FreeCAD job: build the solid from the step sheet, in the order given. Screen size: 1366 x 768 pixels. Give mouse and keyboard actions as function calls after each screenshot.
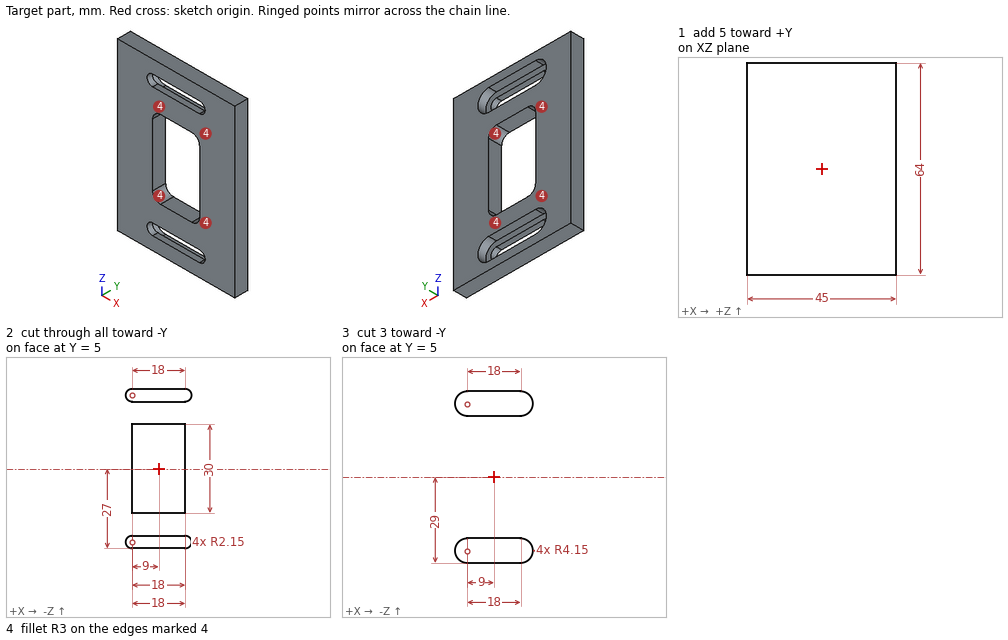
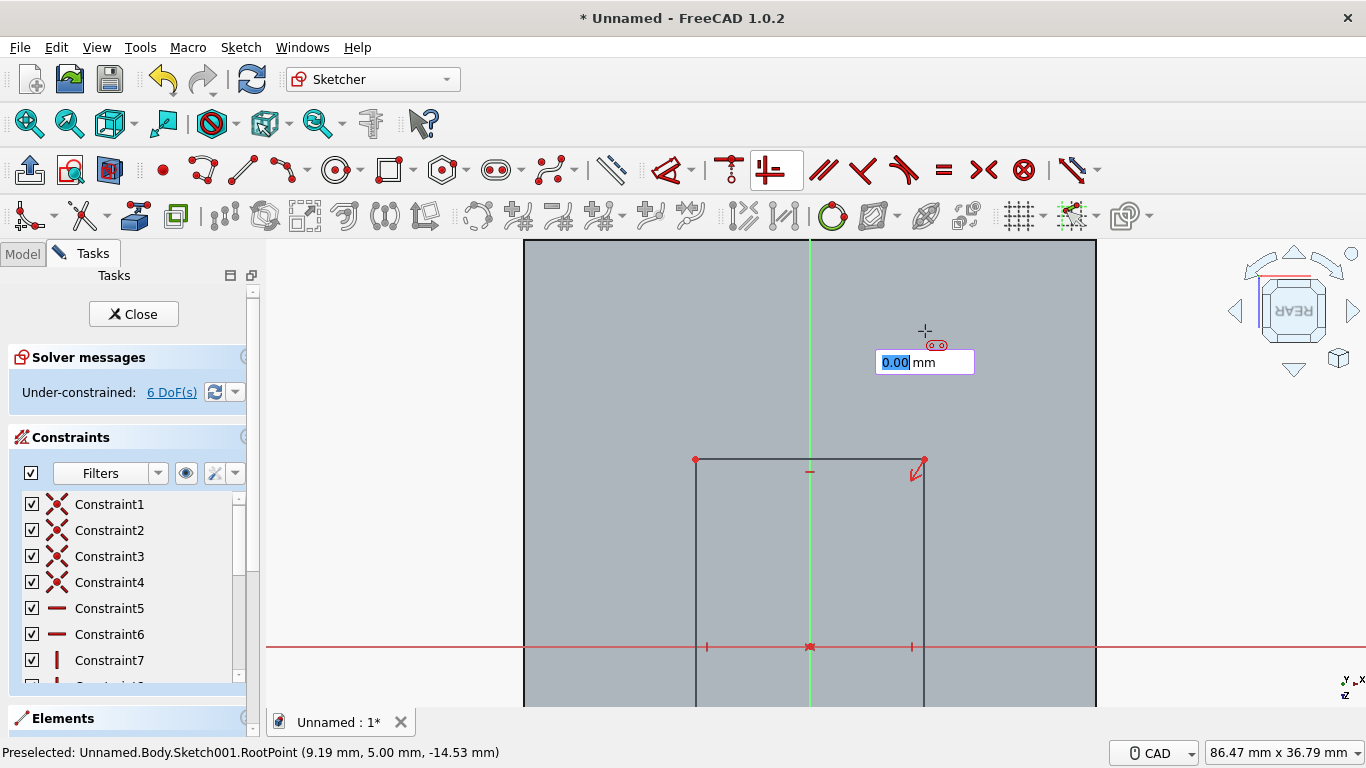
click(776, 358)
key(Escape)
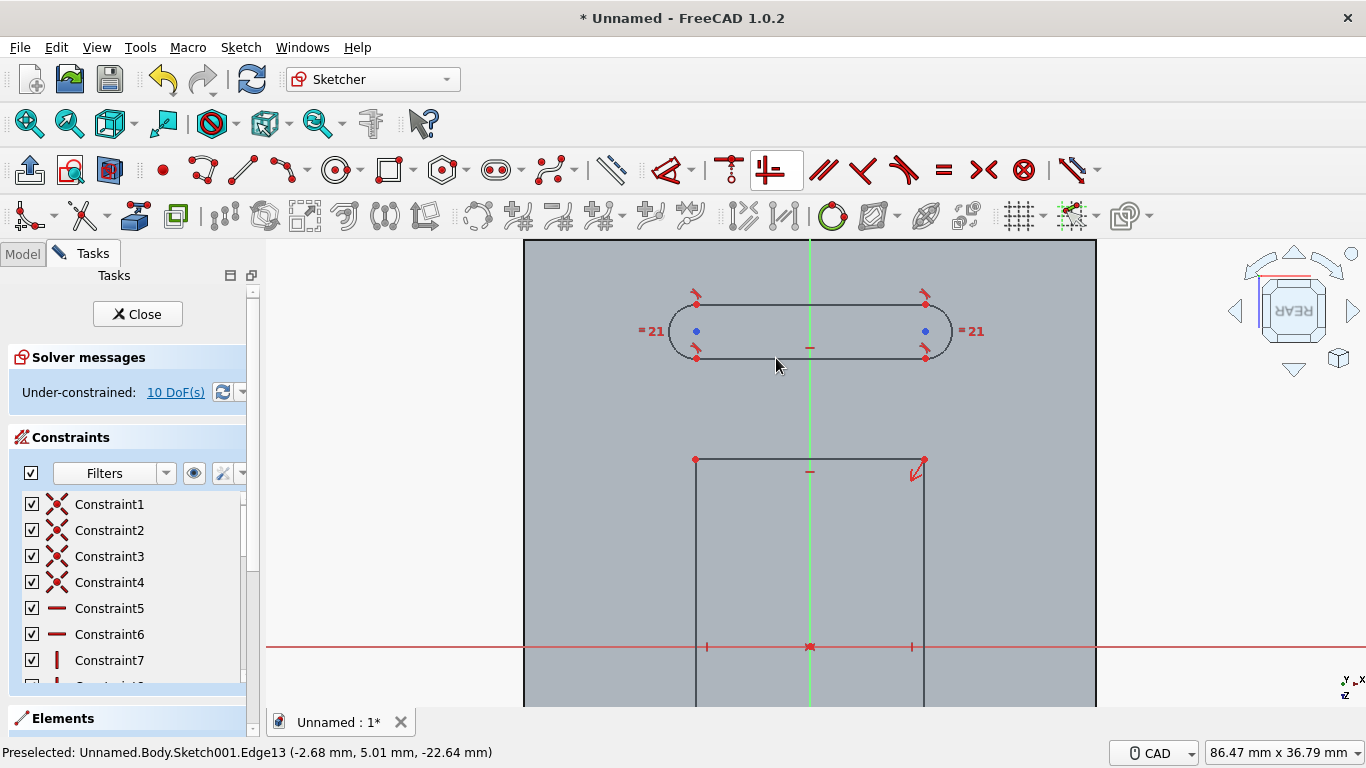
scroll(696, 331, down, 4)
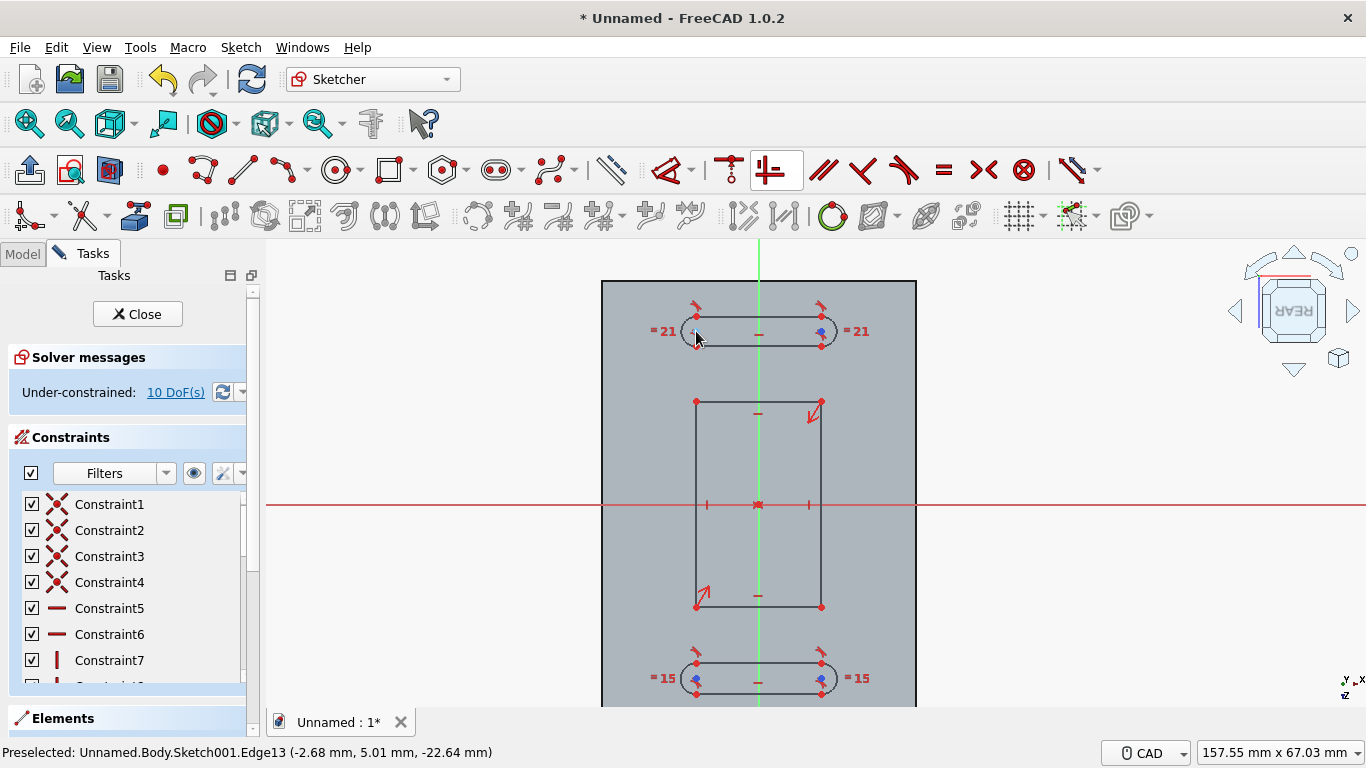
click(686, 608)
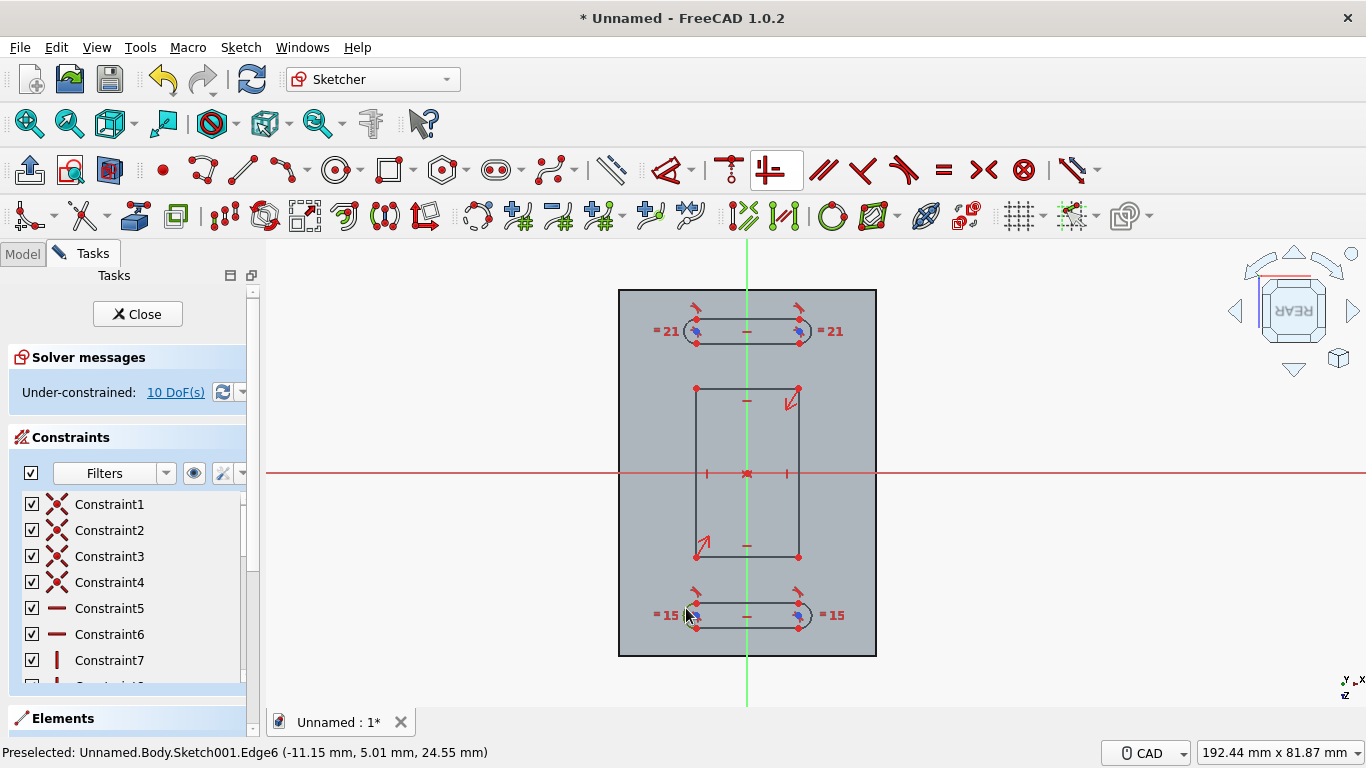
scroll(686, 324, up, 2)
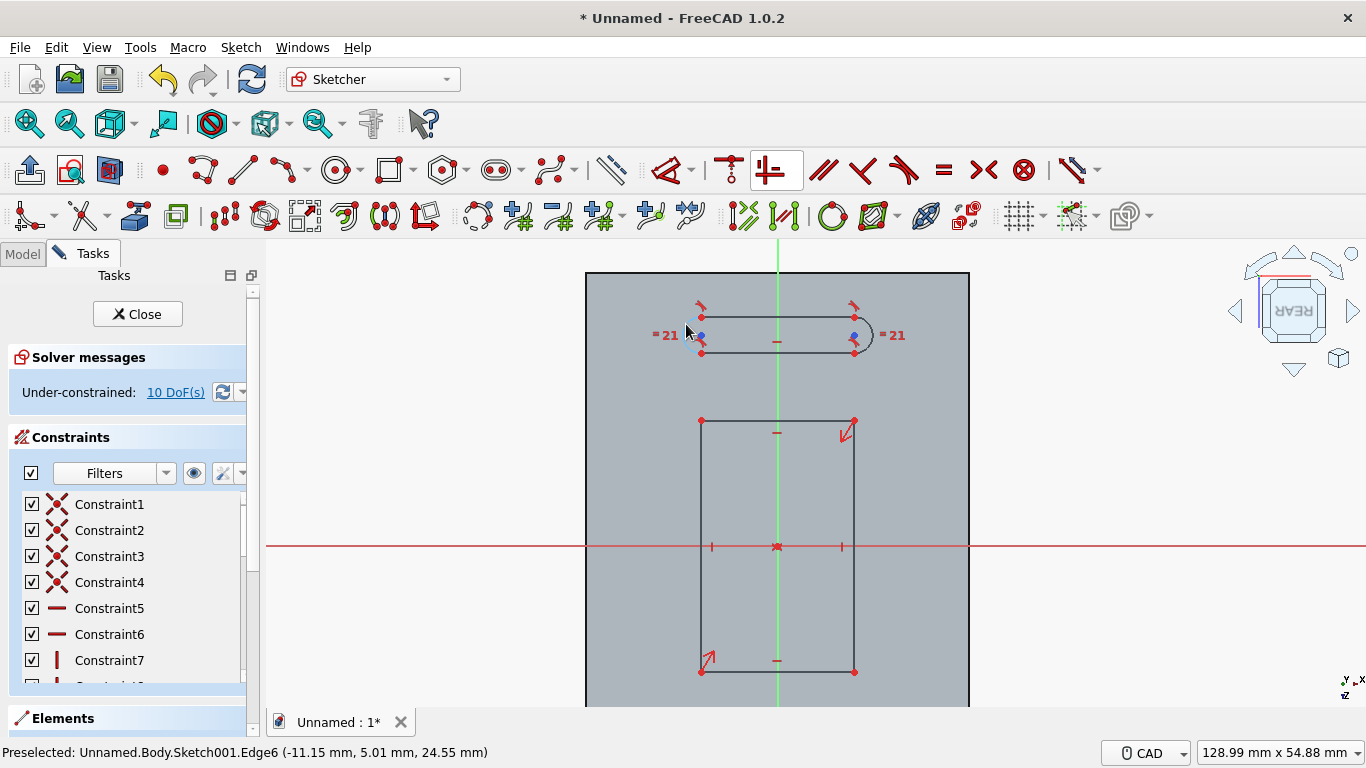
click(686, 325)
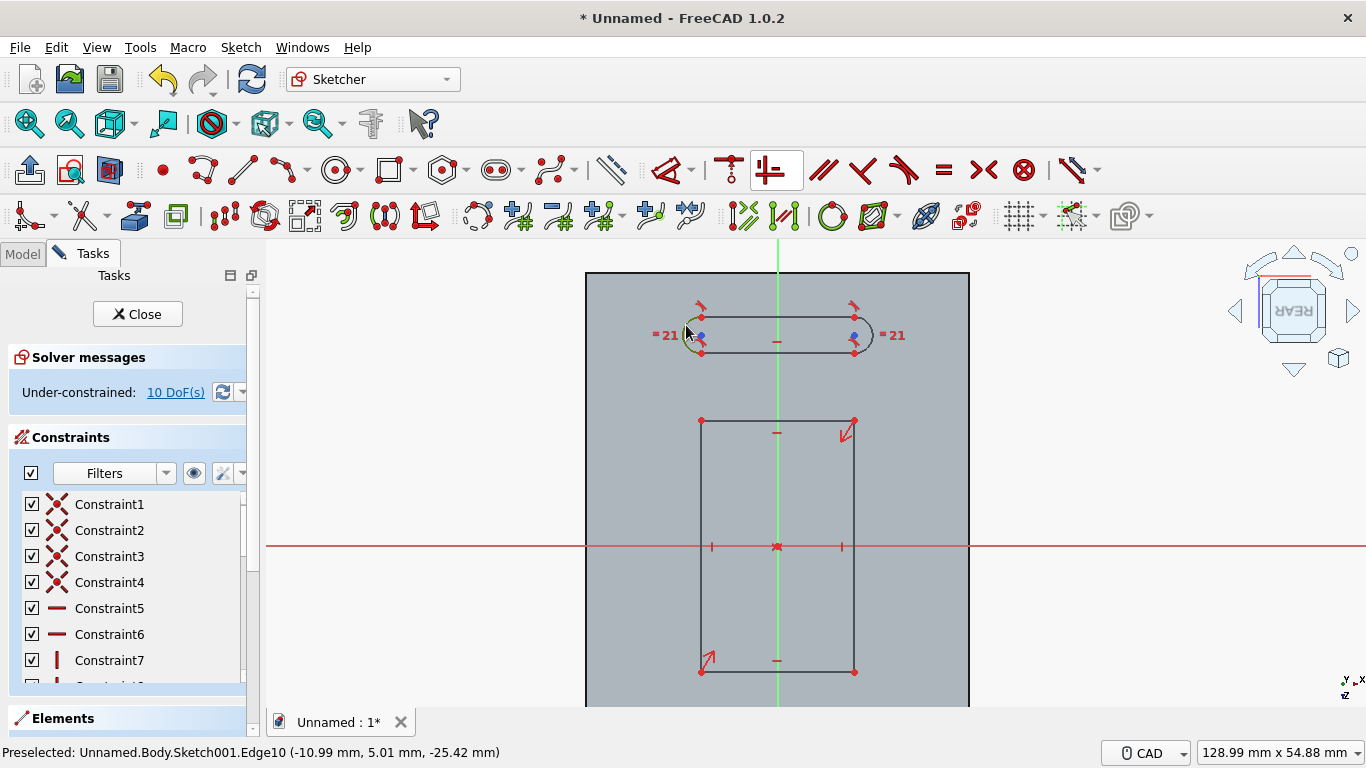
click(944, 170)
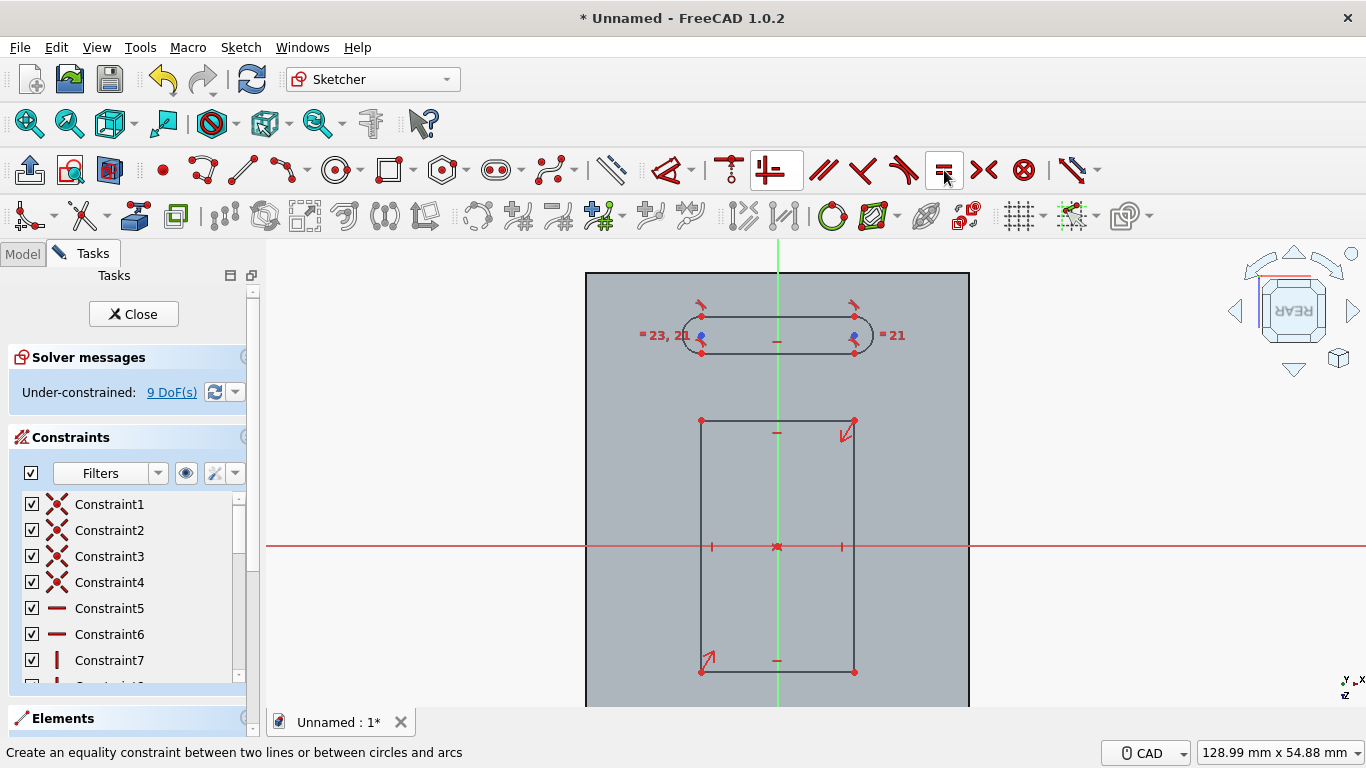
scroll(686, 324, down, 2)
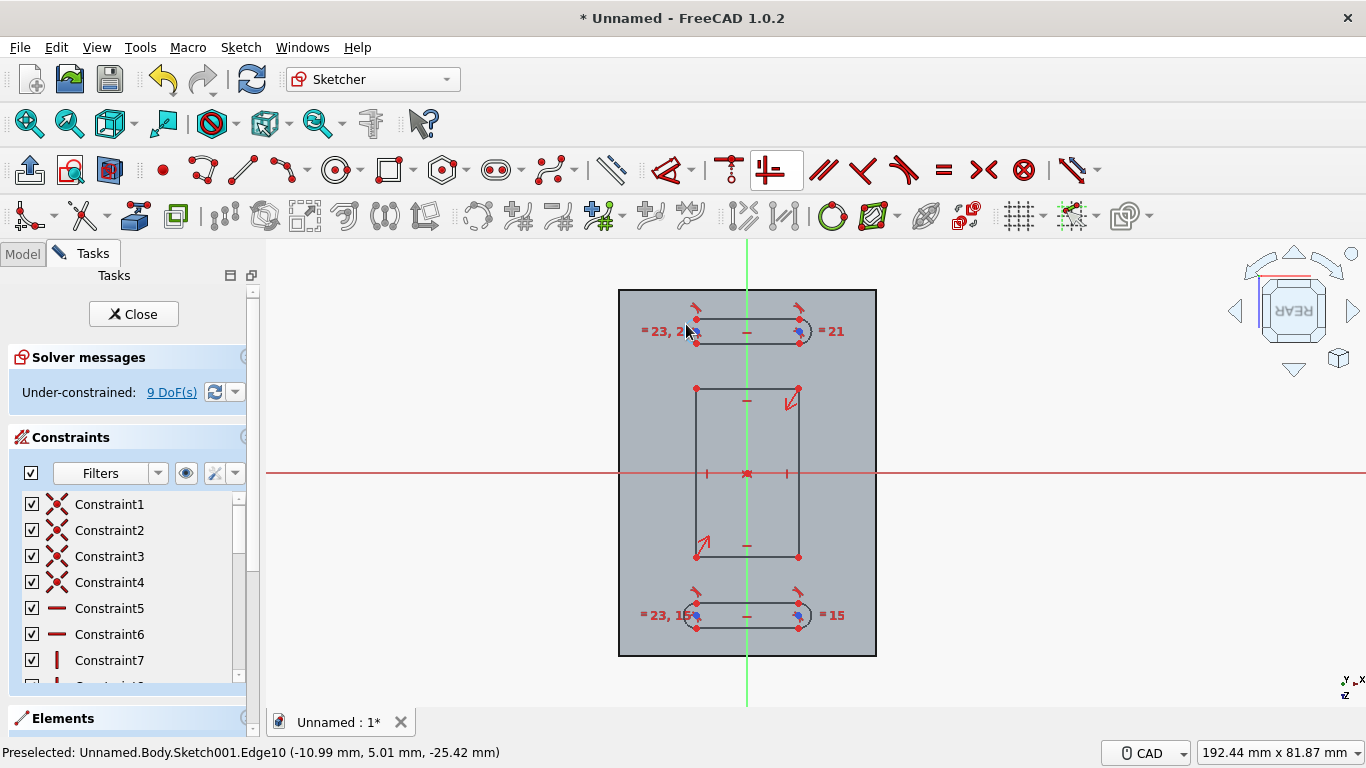
click(696, 616)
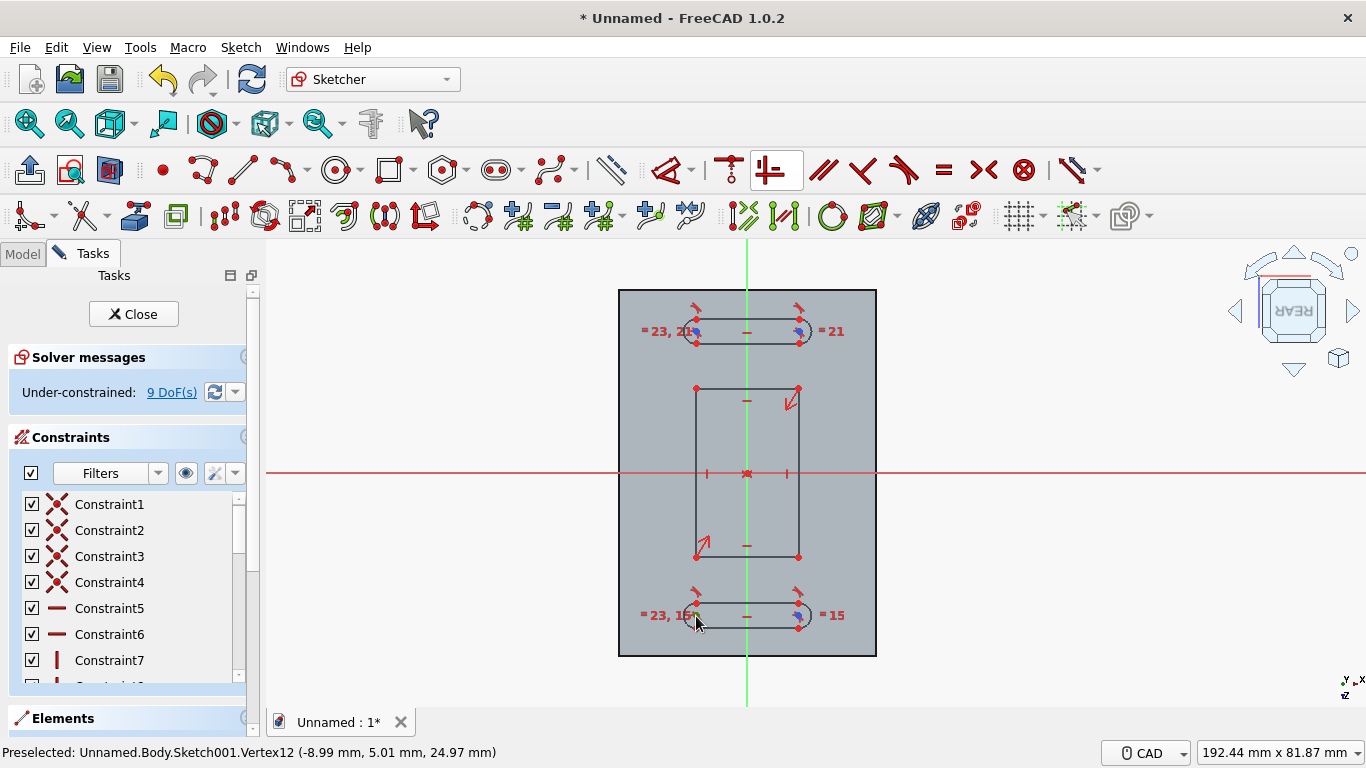
click(696, 332)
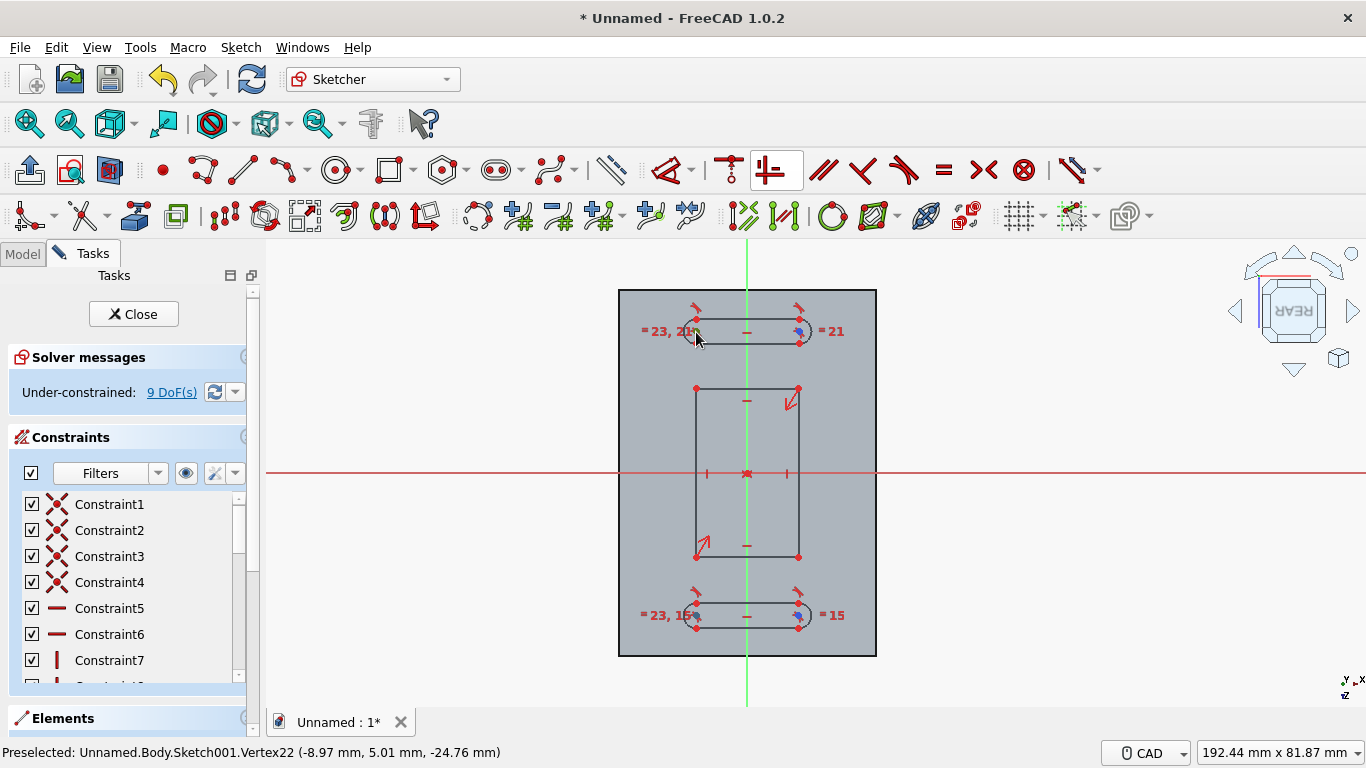
click(359, 473)